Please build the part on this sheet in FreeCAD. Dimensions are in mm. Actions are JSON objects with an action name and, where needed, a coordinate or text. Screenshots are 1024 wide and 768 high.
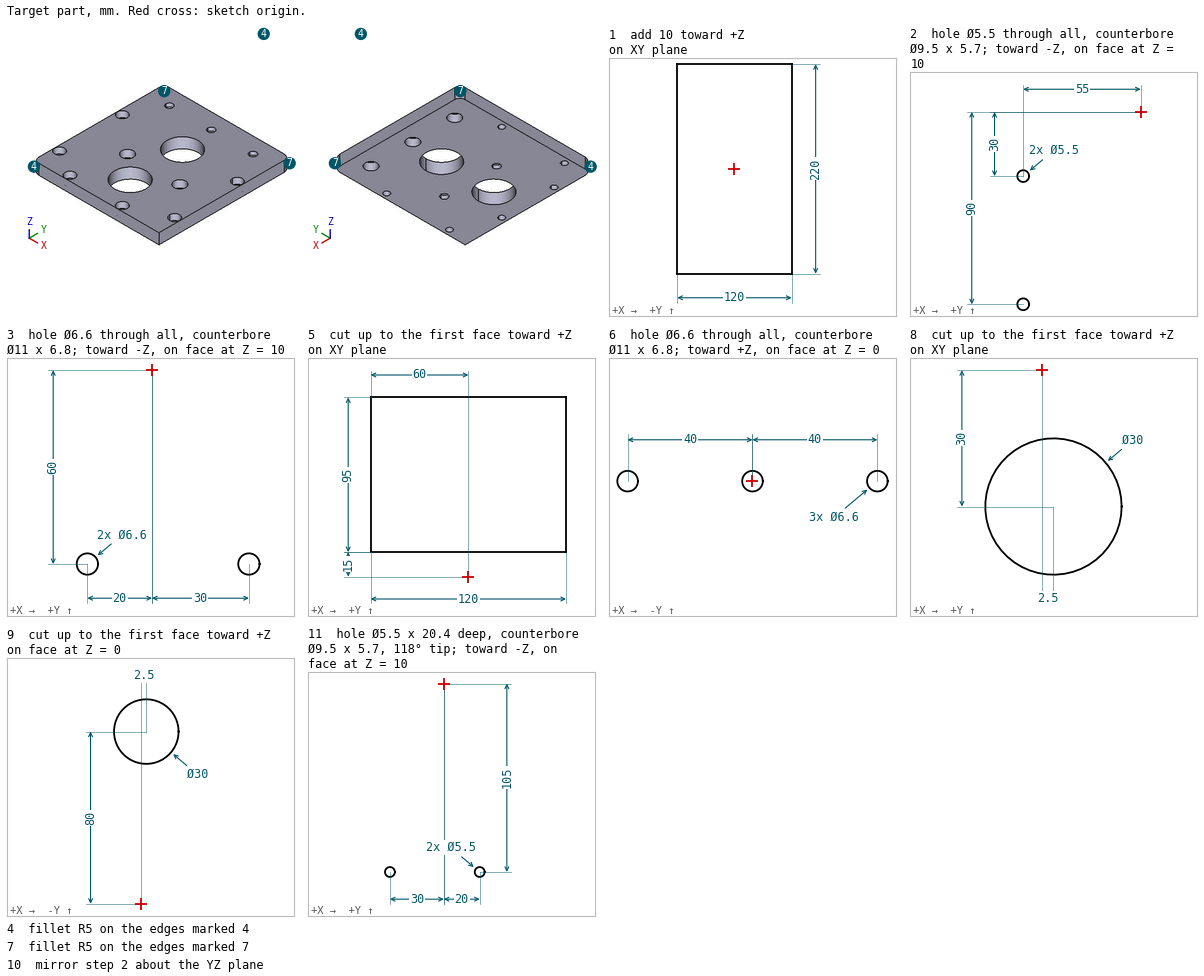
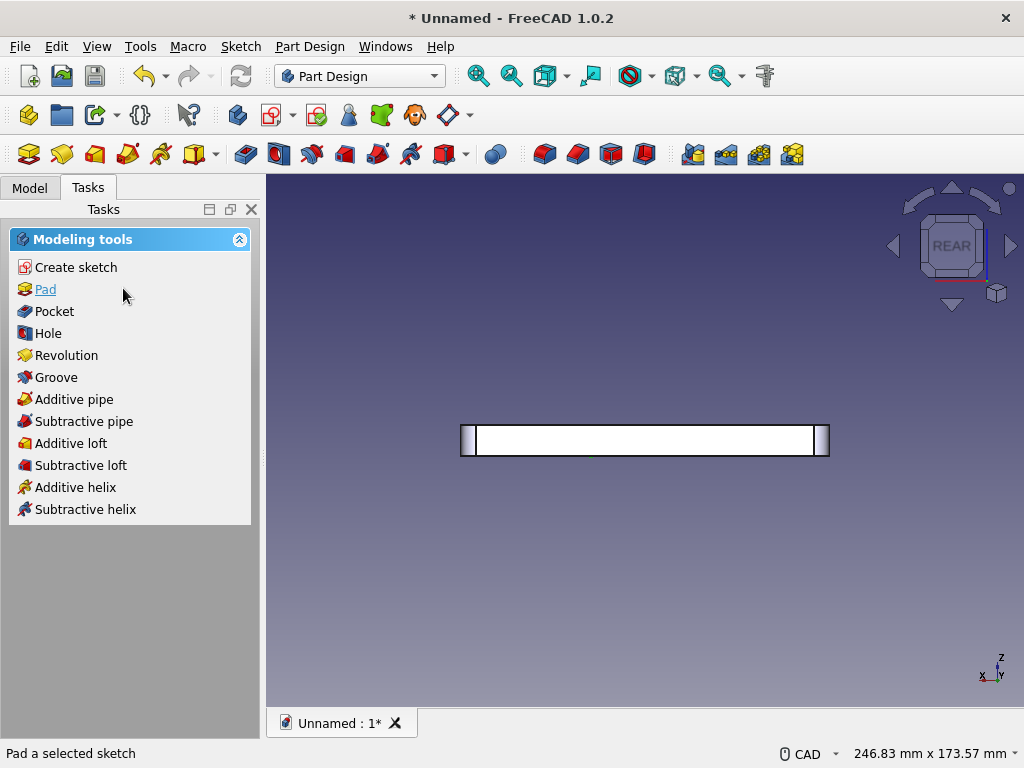
{"action": "left_click", "coordinate": [246, 154]}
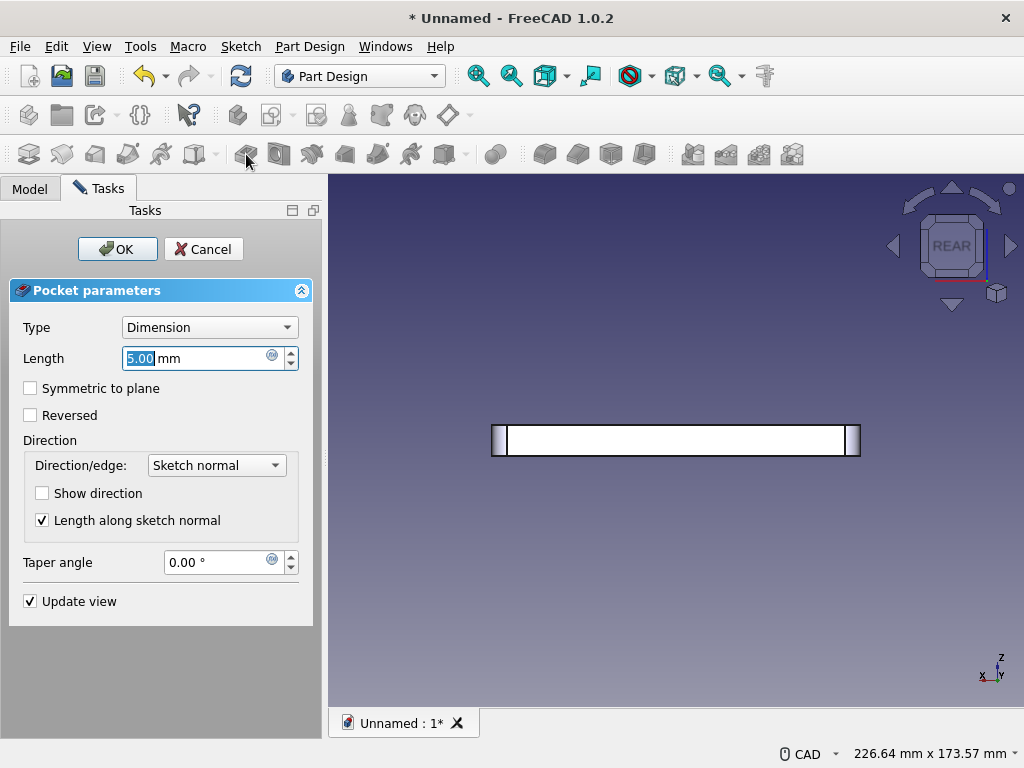
{"action": "left_click", "coordinate": [210, 328]}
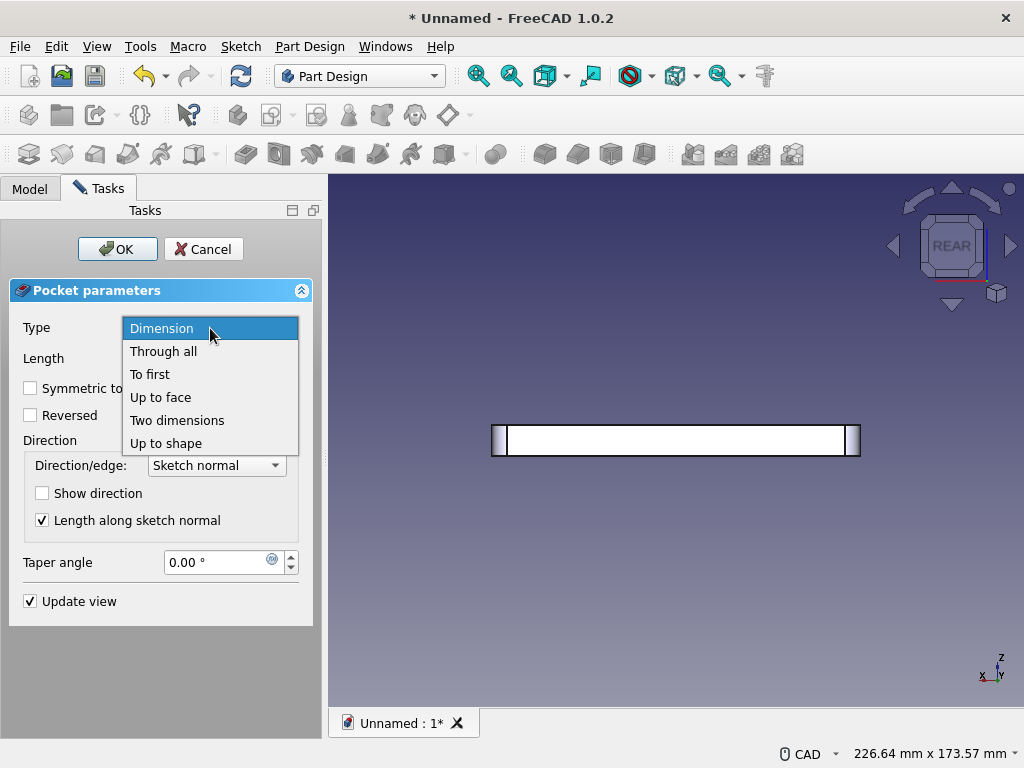
{"action": "left_click", "coordinate": [208, 374]}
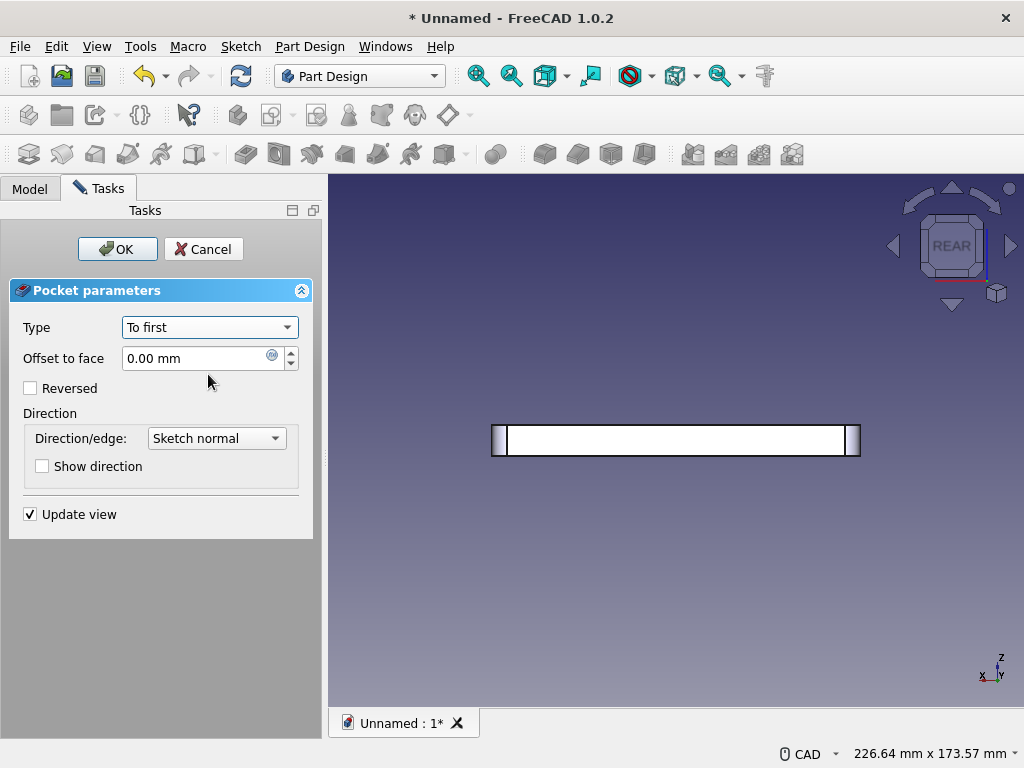
{"action": "left_click", "coordinate": [31, 388]}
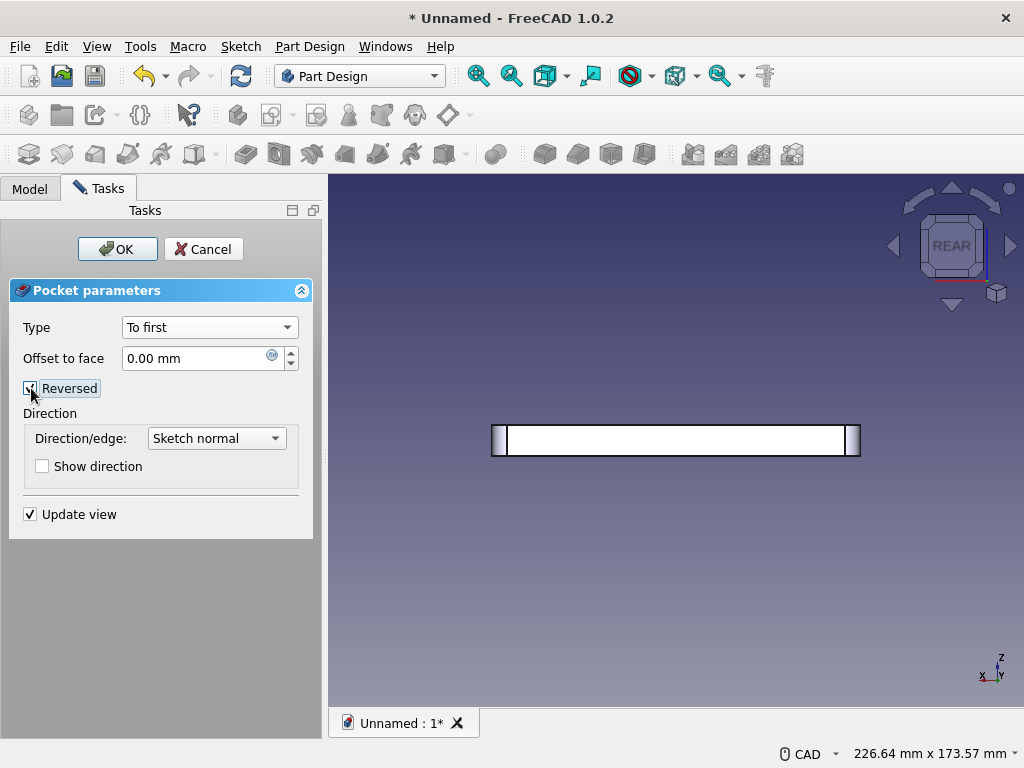
{"action": "left_click", "coordinate": [118, 249]}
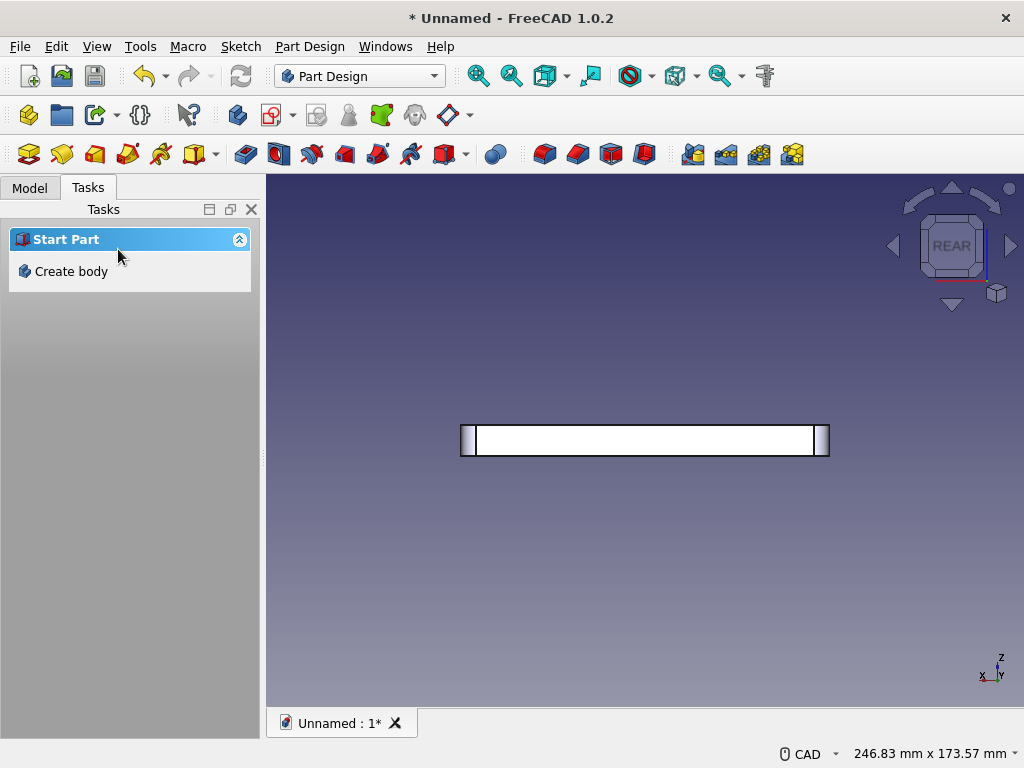
{"action": "key", "text": "5"}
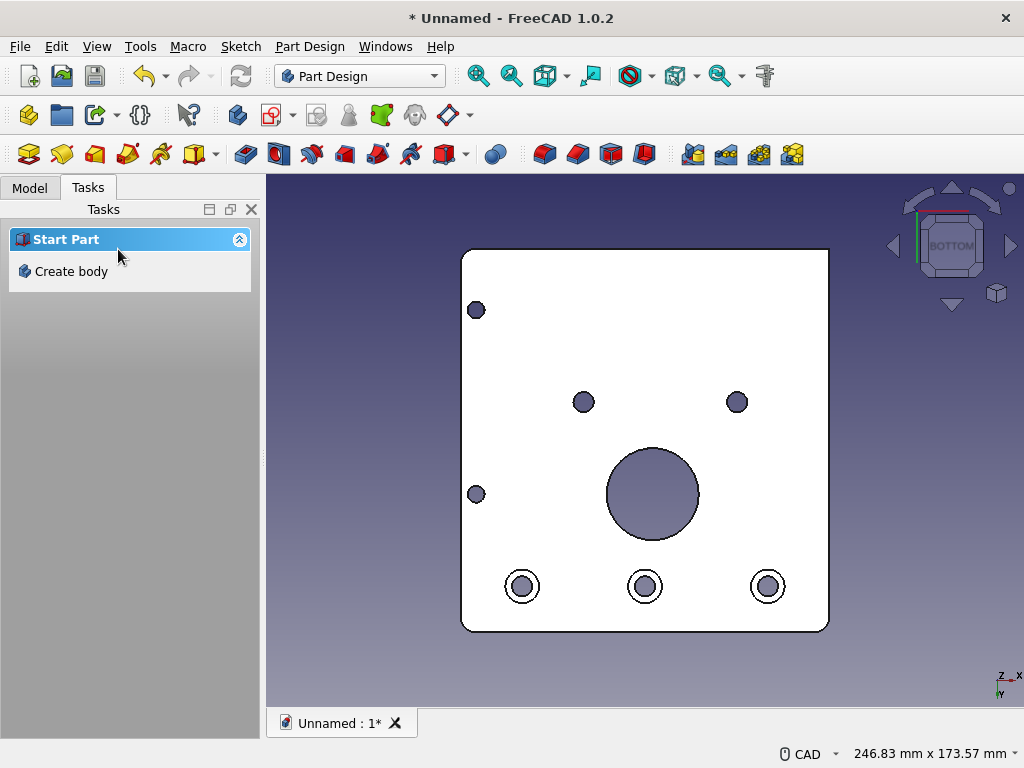
{"action": "left_click", "coordinate": [645, 330]}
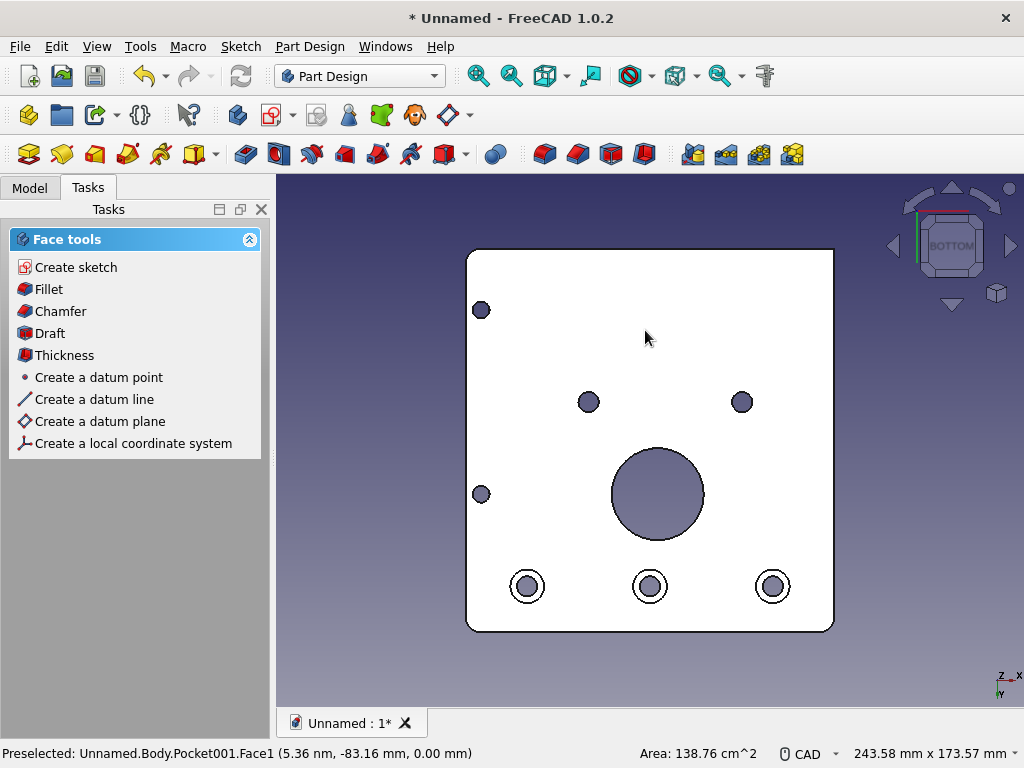
{"action": "left_click", "coordinate": [270, 116]}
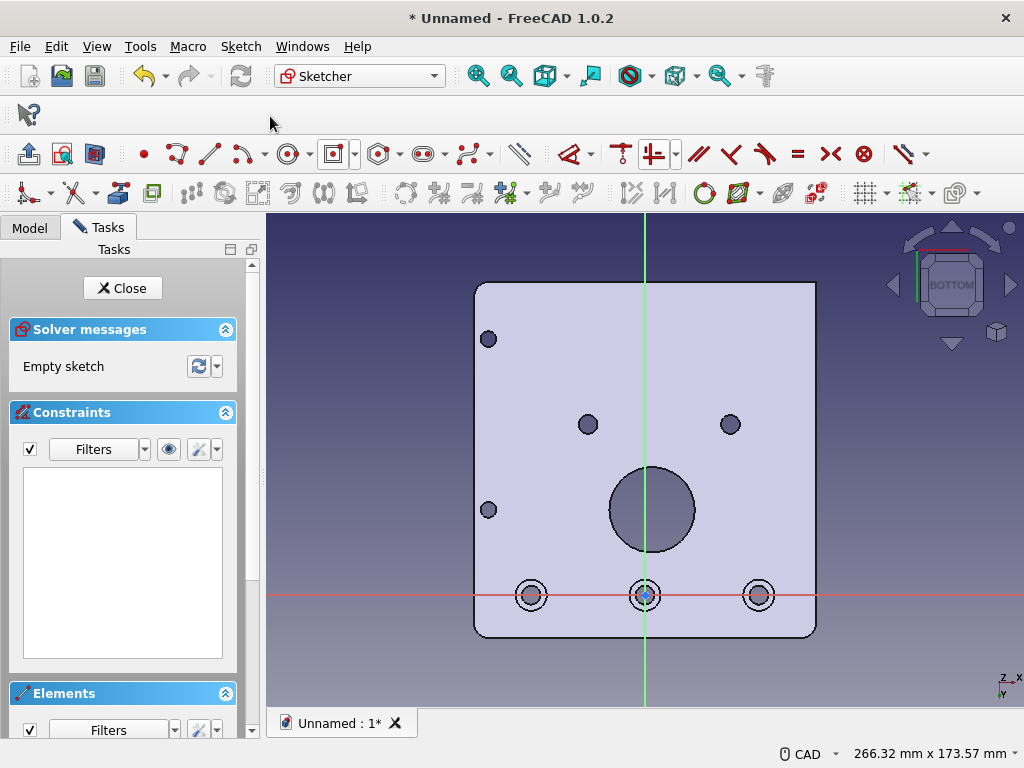
{"action": "scroll", "coordinate": [685, 328], "scroll_direction": "up", "scroll_amount": 6}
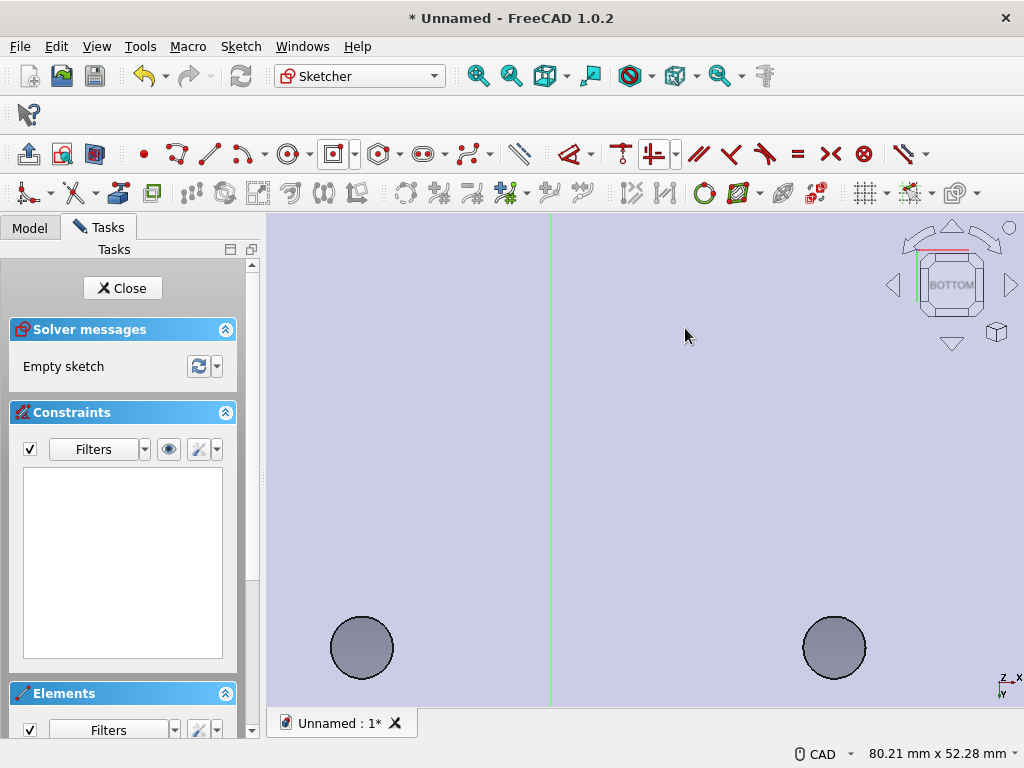
{"action": "left_click", "coordinate": [288, 154]}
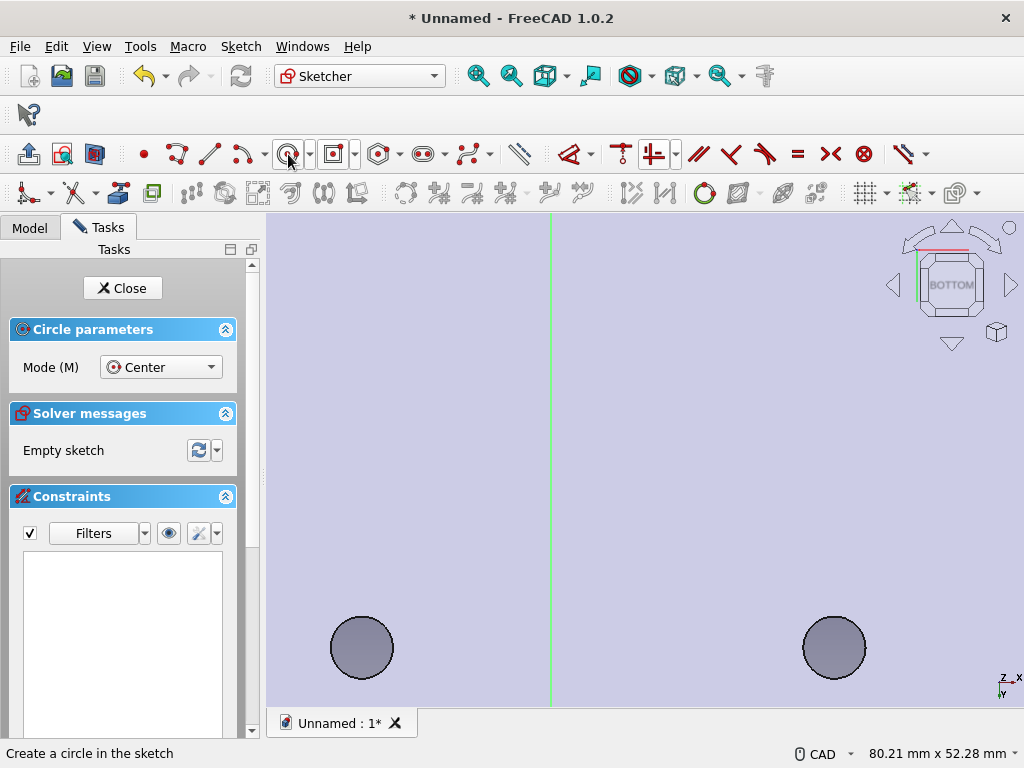
{"action": "left_click", "coordinate": [575, 459]}
{"action": "left_click", "coordinate": [675, 358]}
{"action": "key", "text": "Escape"}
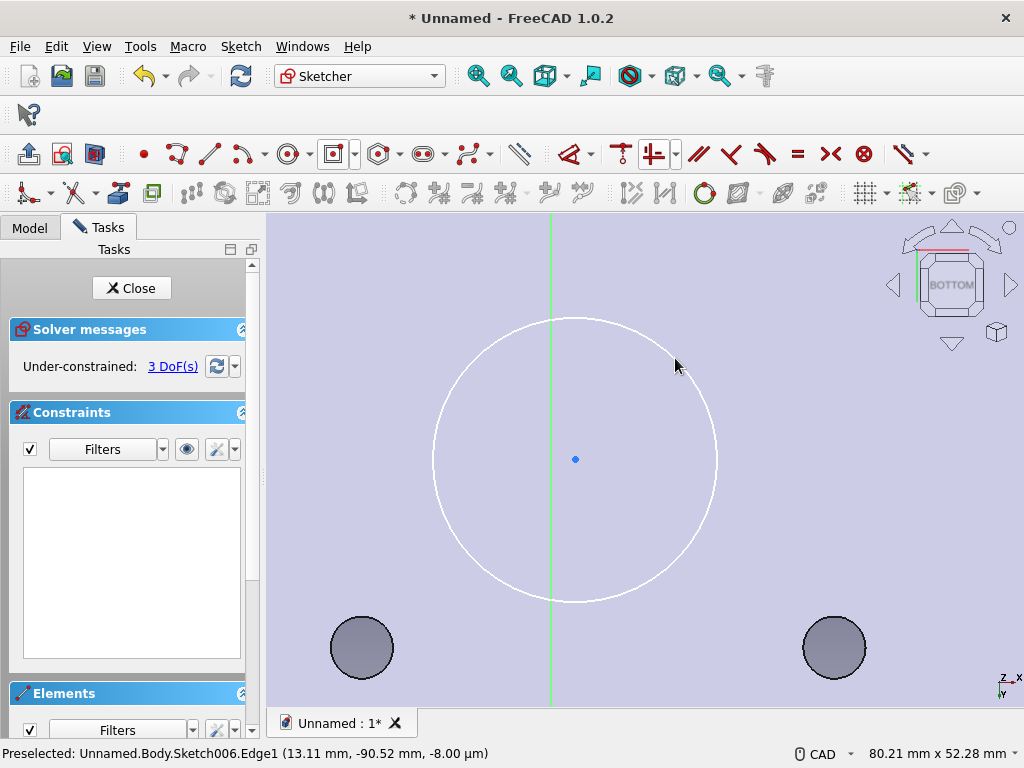
{"action": "left_click", "coordinate": [568, 154]}